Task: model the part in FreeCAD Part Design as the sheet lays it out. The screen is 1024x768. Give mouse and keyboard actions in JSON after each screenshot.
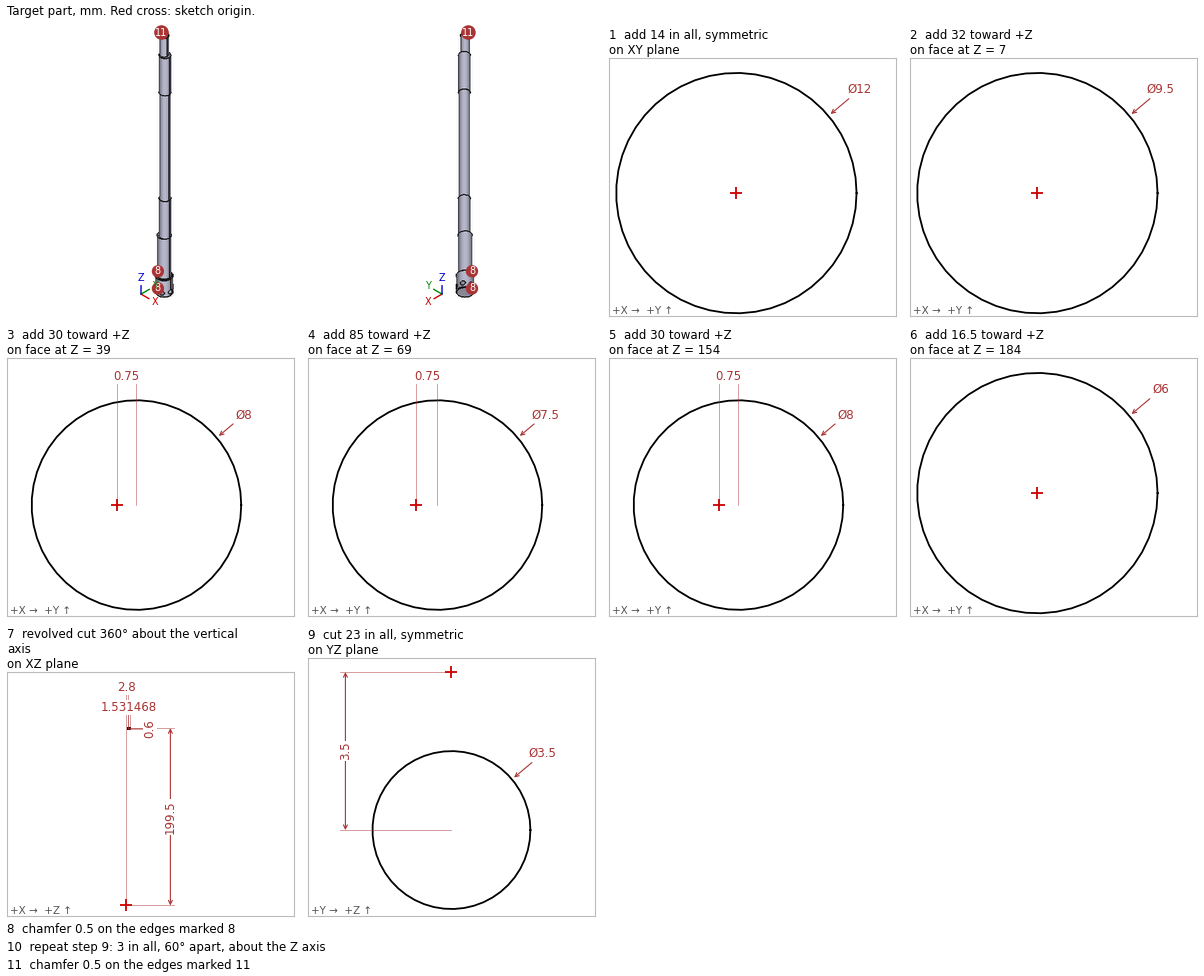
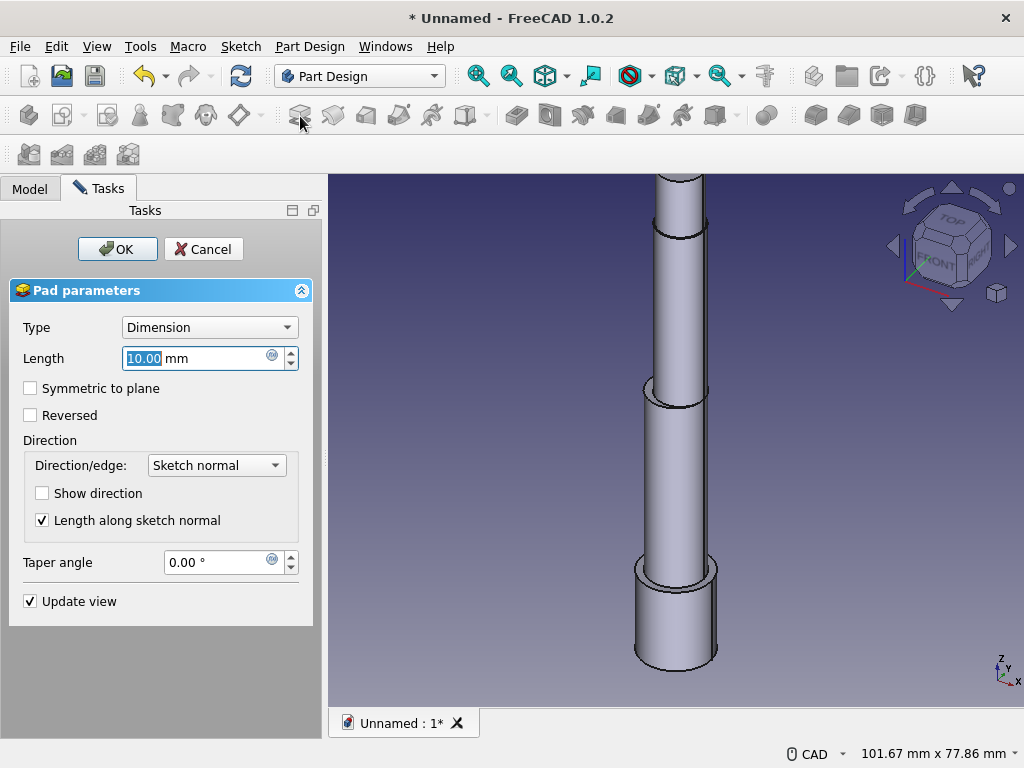
{"action": "type", "text": "85"}
{"action": "key", "text": "Tab"}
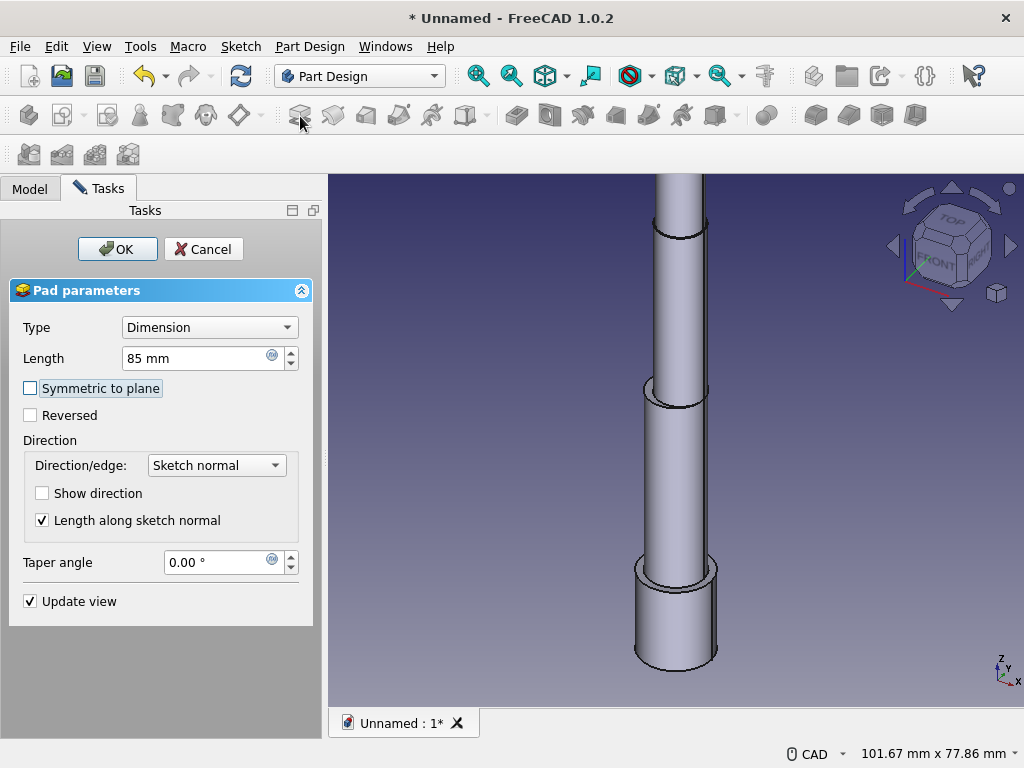
{"action": "left_click", "coordinate": [118, 249]}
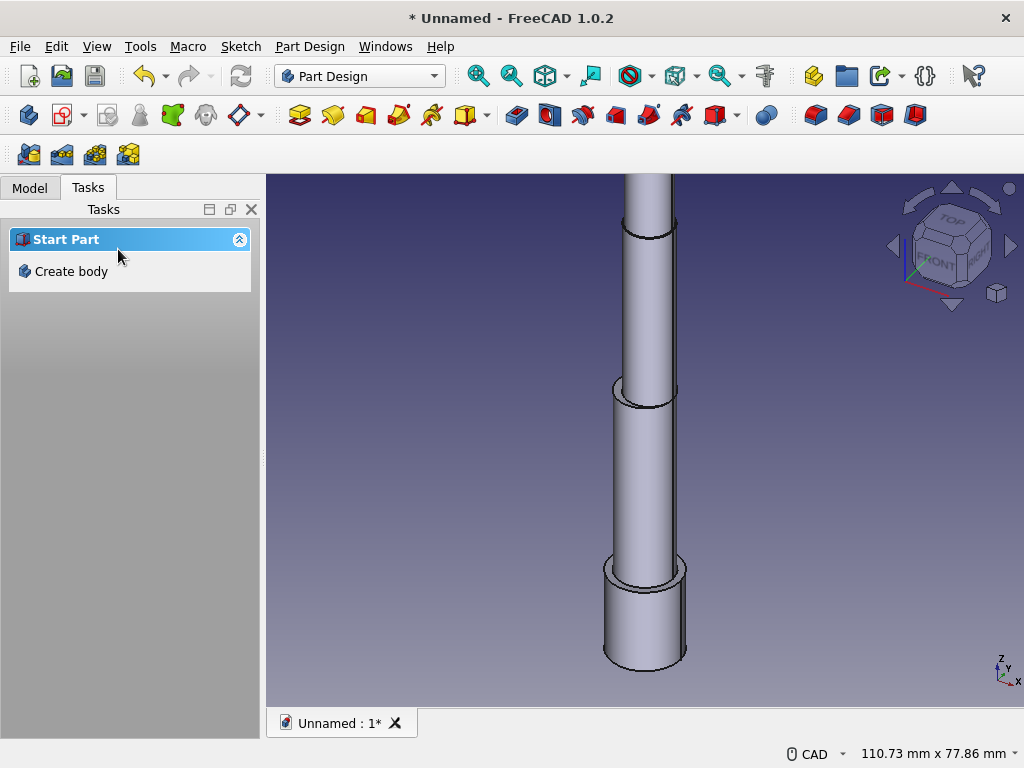
{"action": "key", "text": "v f"}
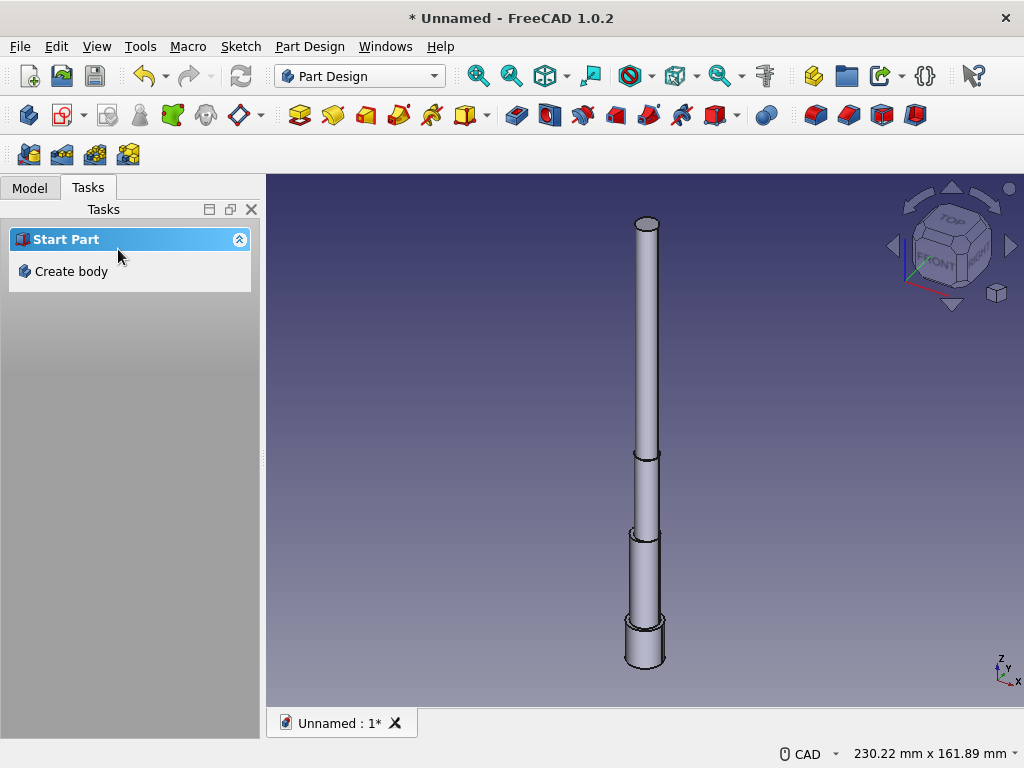
{"action": "left_click", "coordinate": [649, 221]}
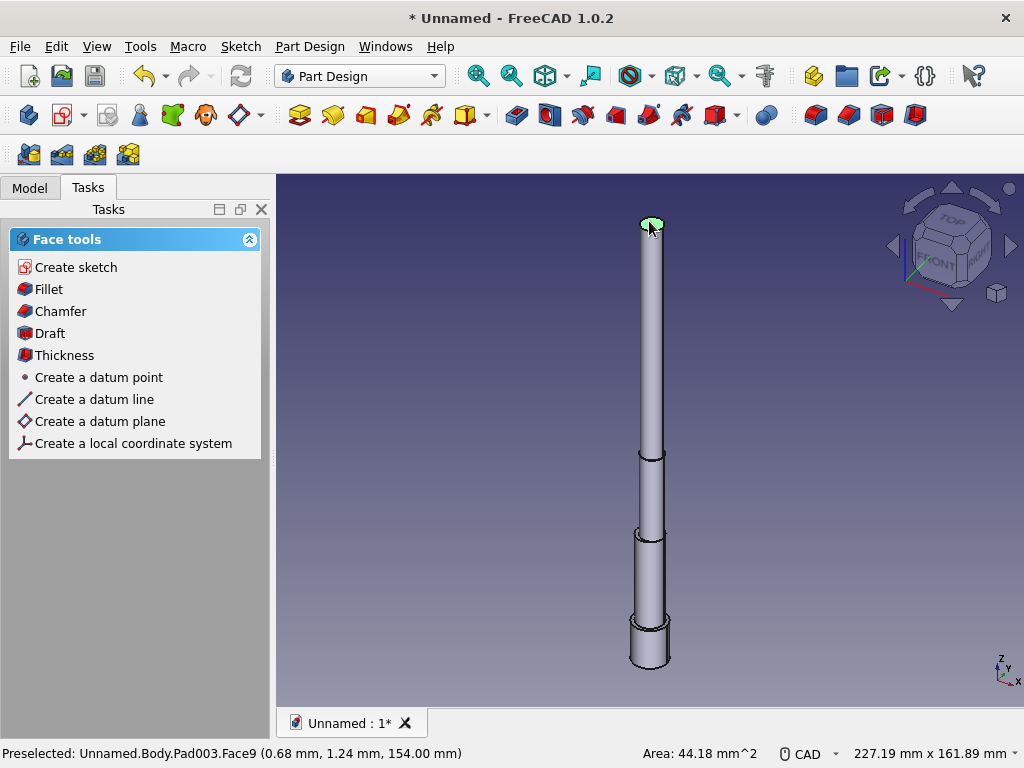
{"action": "left_click", "coordinate": [62, 116]}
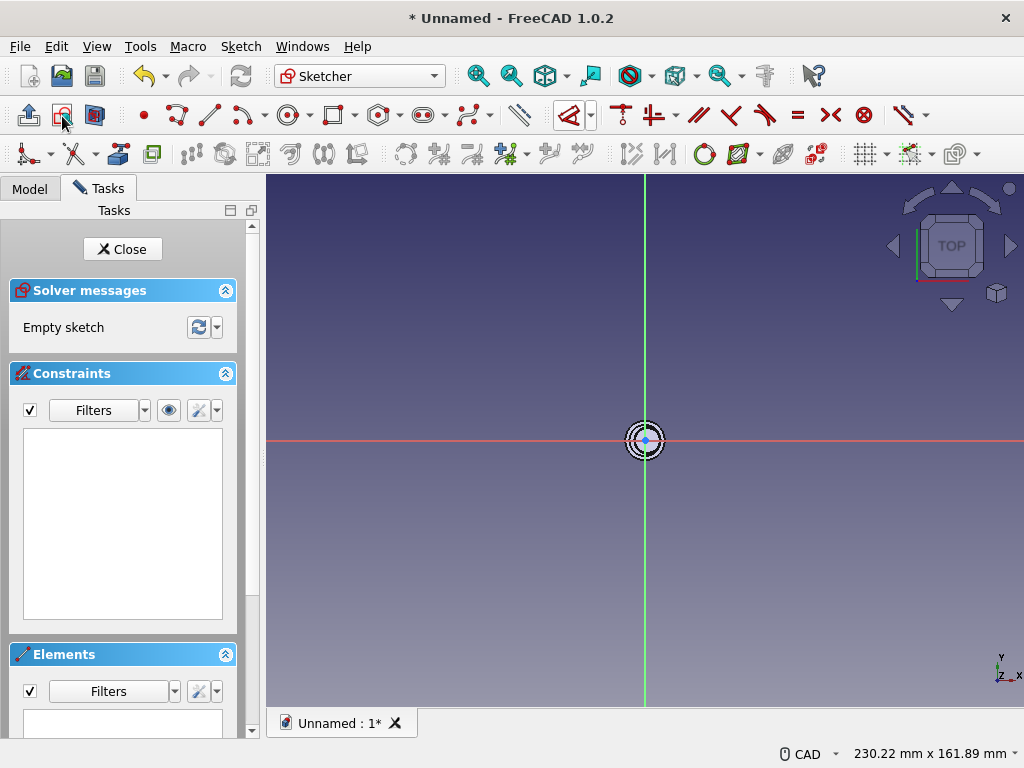
{"action": "scroll", "coordinate": [653, 440], "scroll_direction": "up", "scroll_amount": 13}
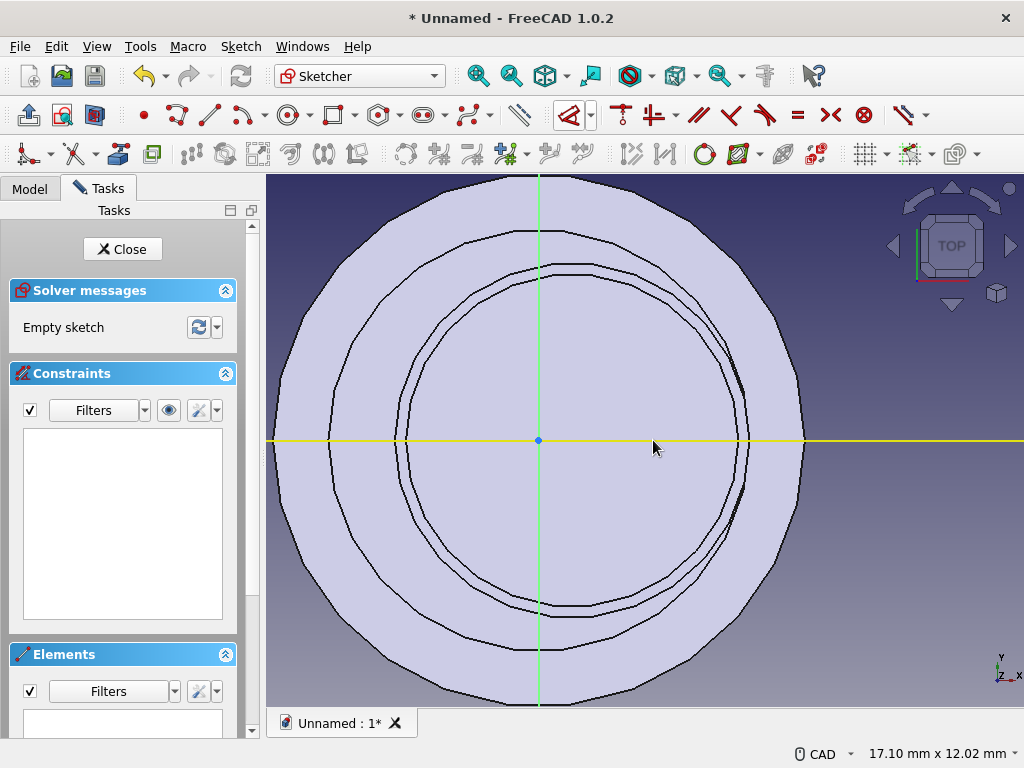
{"action": "key", "text": "g c"}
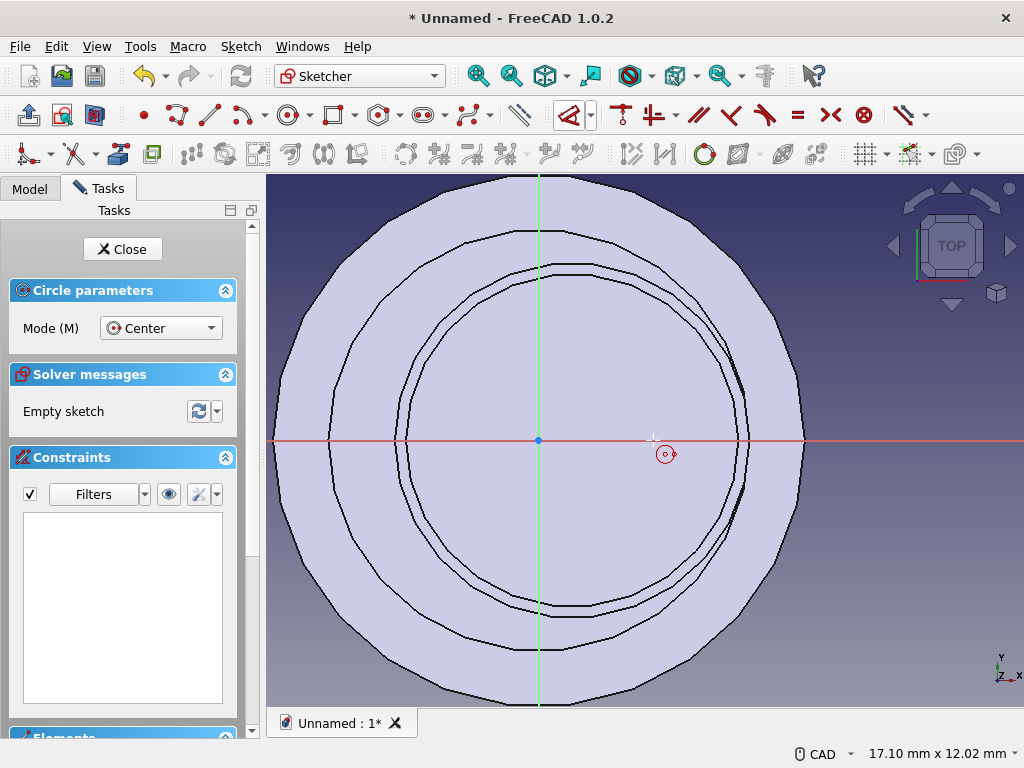
{"action": "left_click", "coordinate": [572, 440]}
{"action": "left_click", "coordinate": [698, 315]}
{"action": "key", "text": "Escape"}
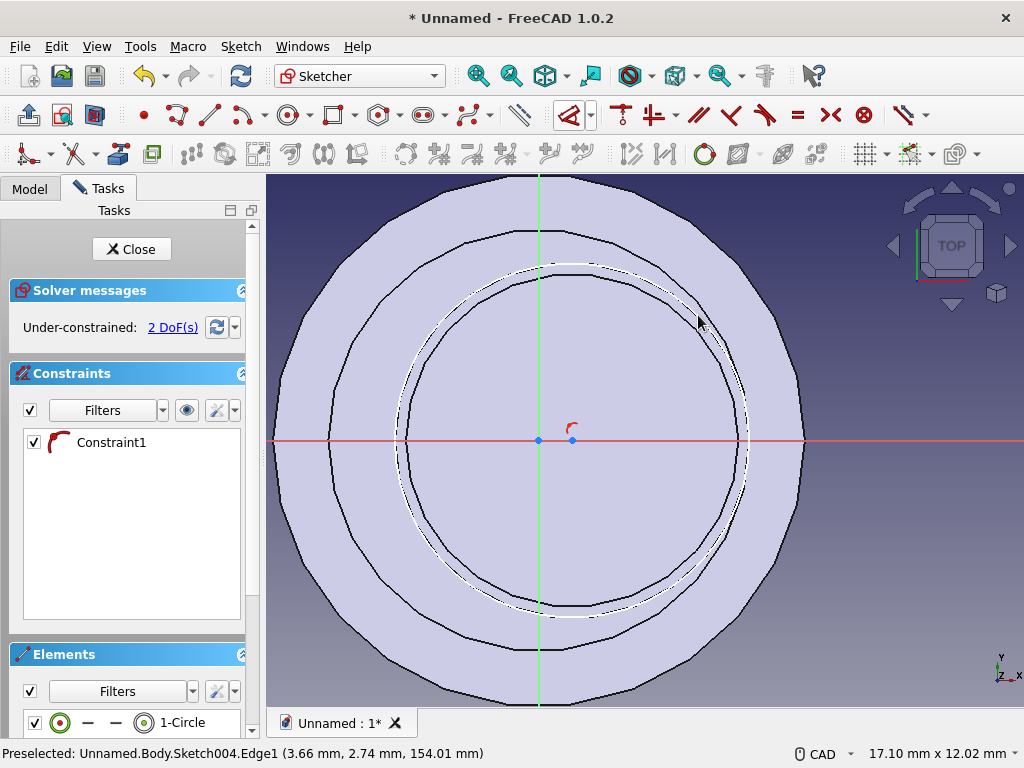
{"action": "left_click", "coordinate": [697, 315]}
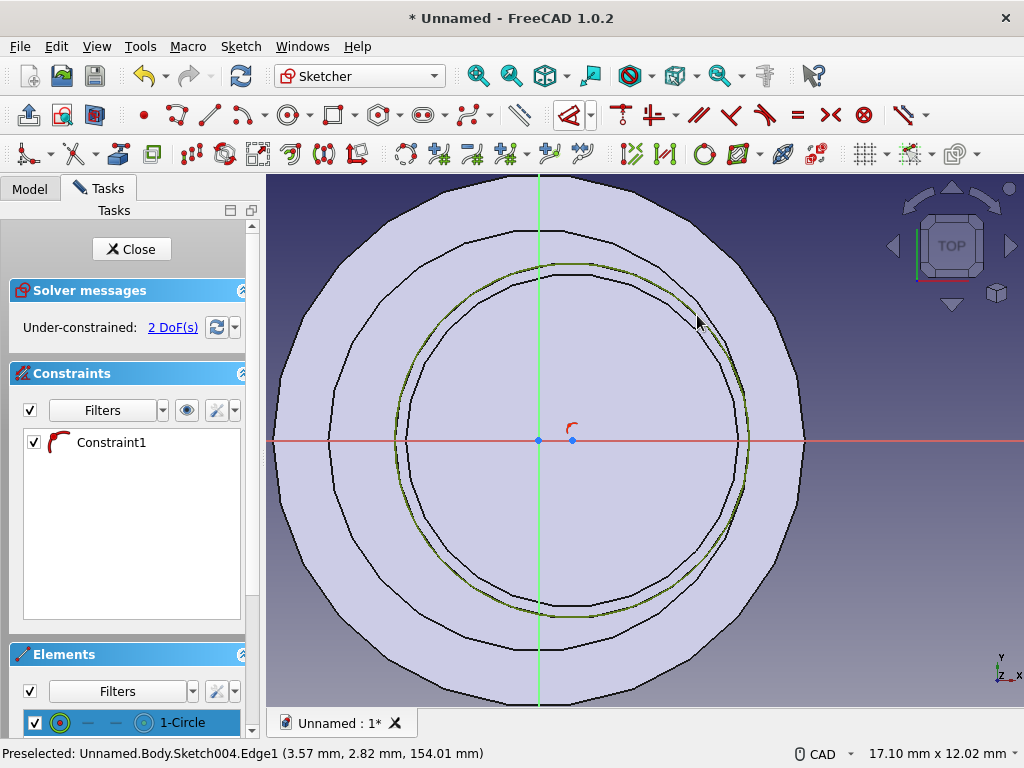
{"action": "key", "text": "k o"}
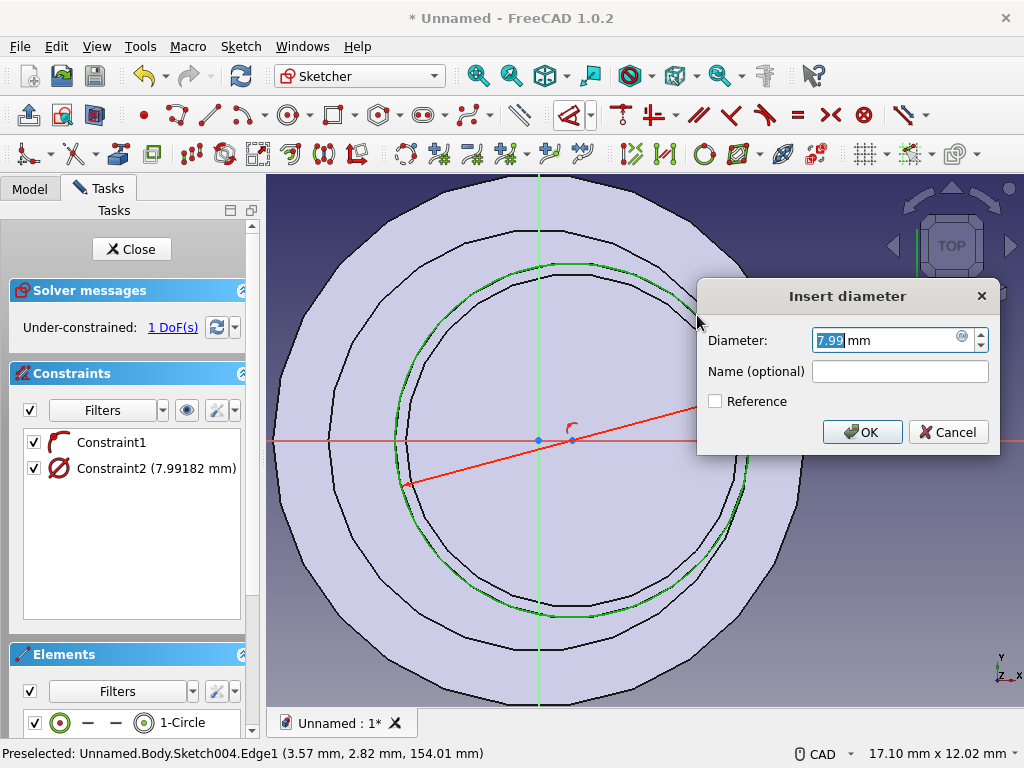
{"action": "type", "text": "8"}
{"action": "key", "text": "Return"}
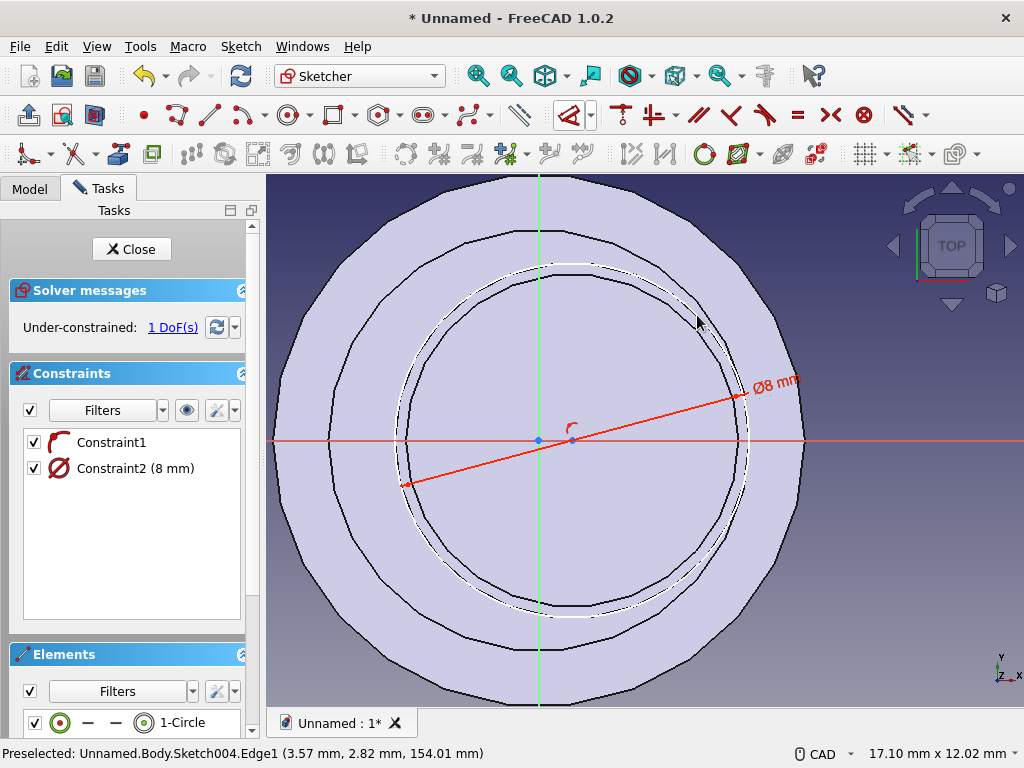
{"action": "scroll", "coordinate": [572, 440], "scroll_direction": "up", "scroll_amount": 4}